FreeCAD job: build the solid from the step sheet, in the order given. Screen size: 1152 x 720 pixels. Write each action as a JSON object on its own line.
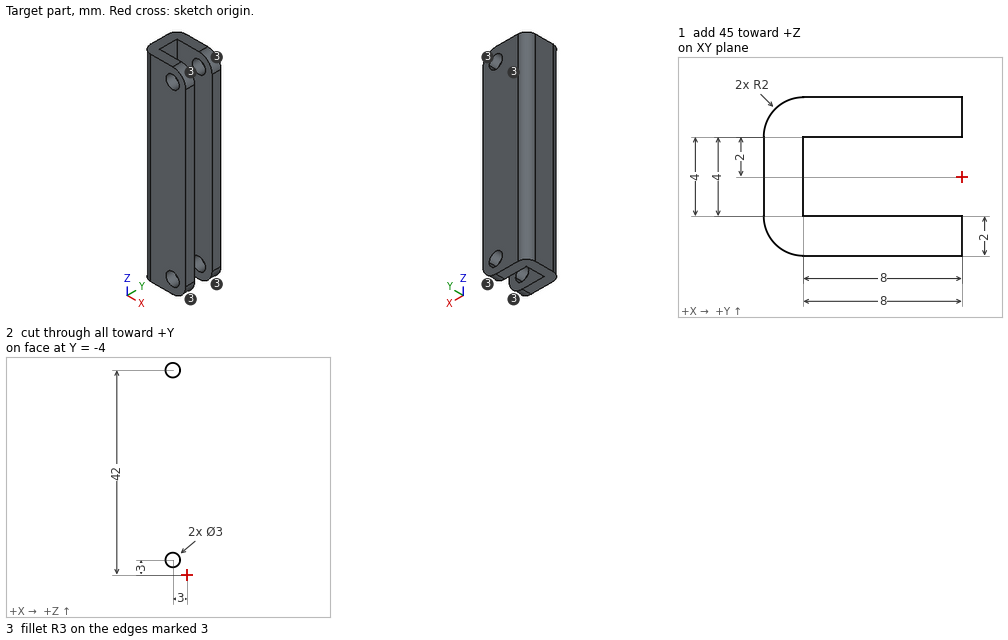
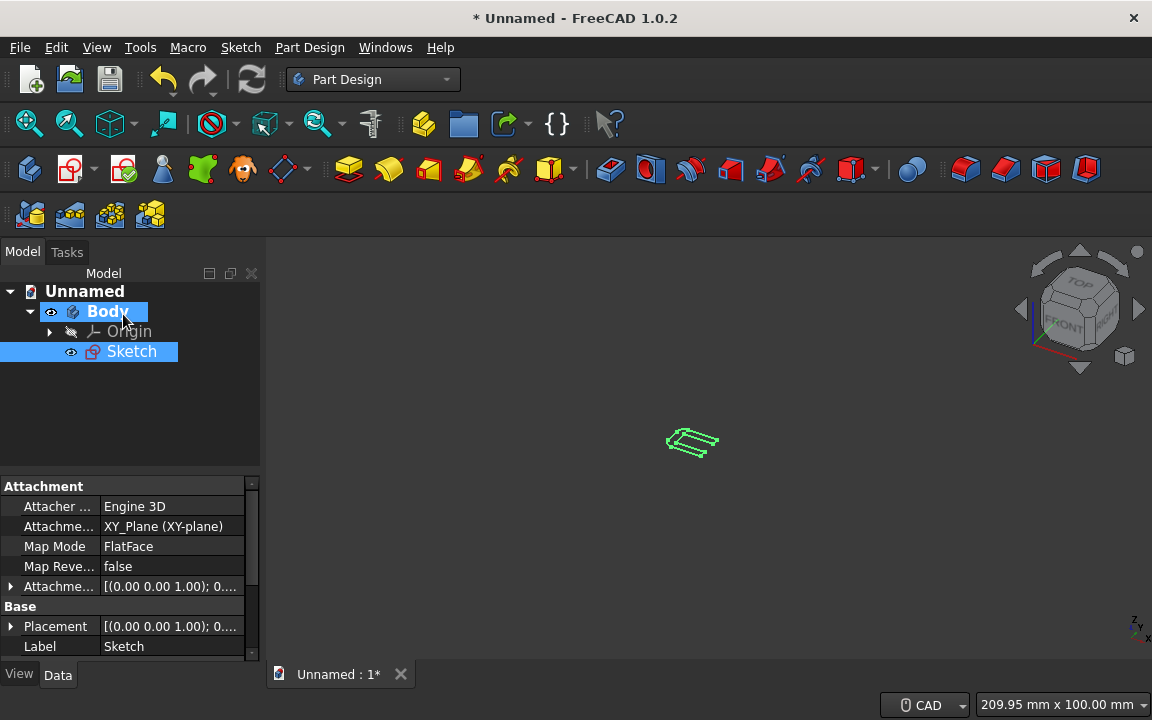
{"action": "left_click", "coordinate": [350, 170]}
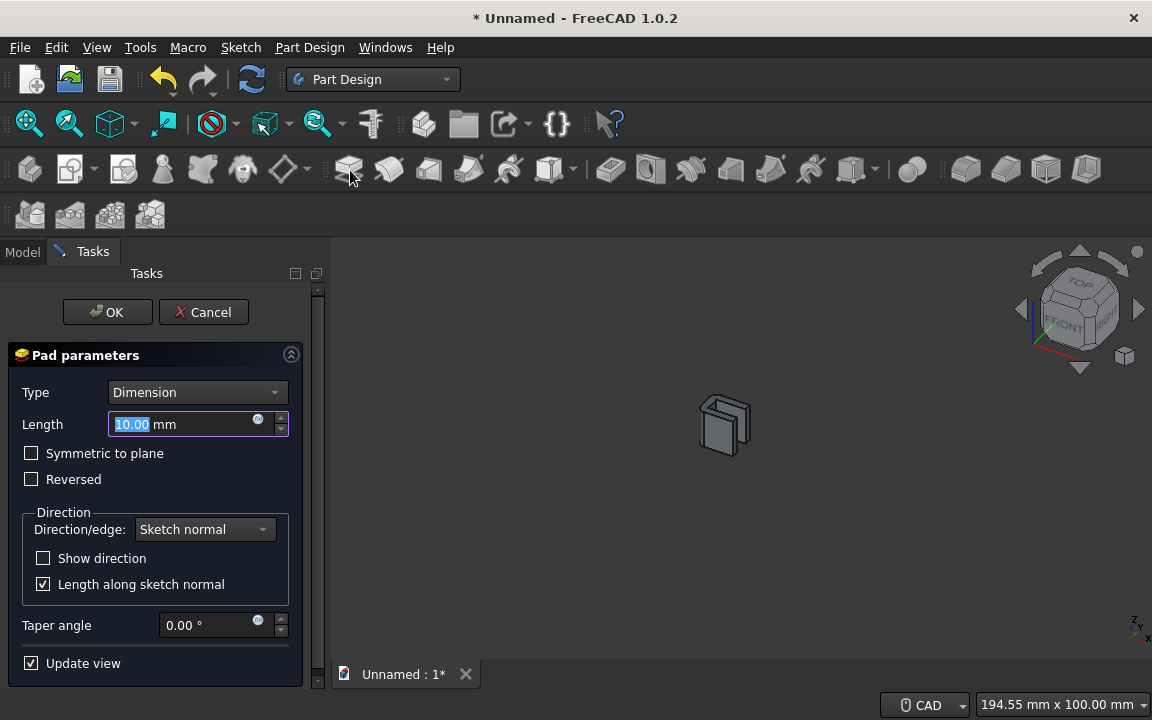
{"action": "type", "text": "45"}
{"action": "key", "text": "Tab"}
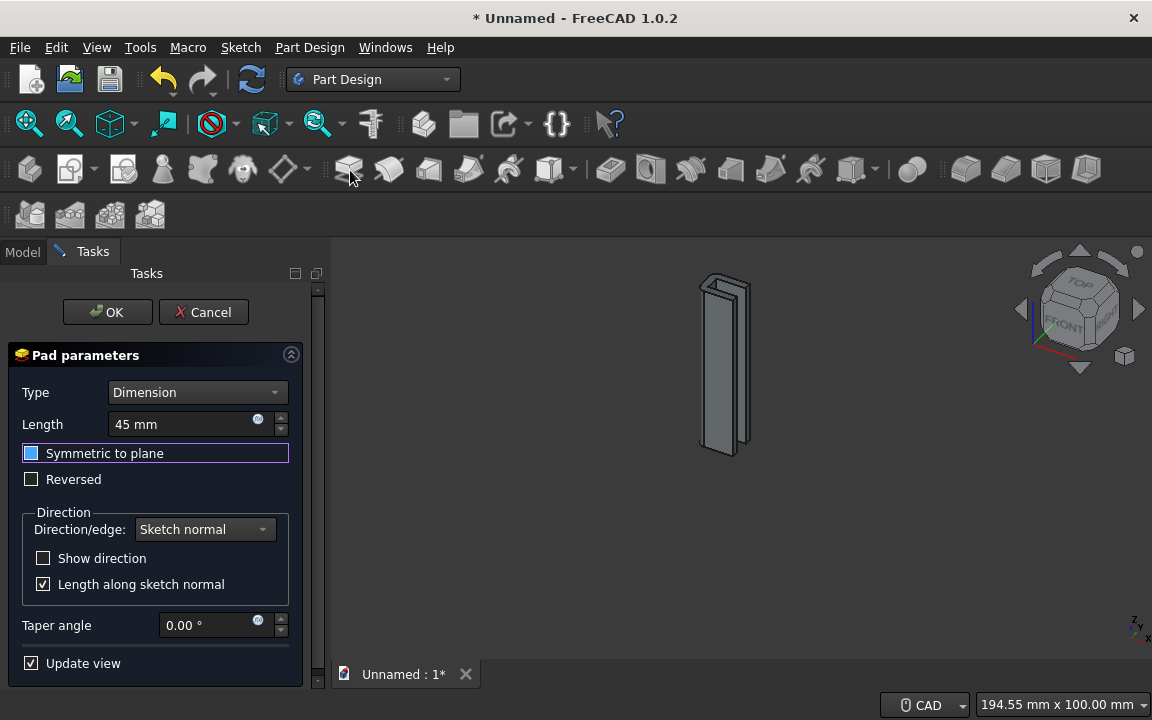
{"action": "left_click", "coordinate": [108, 312]}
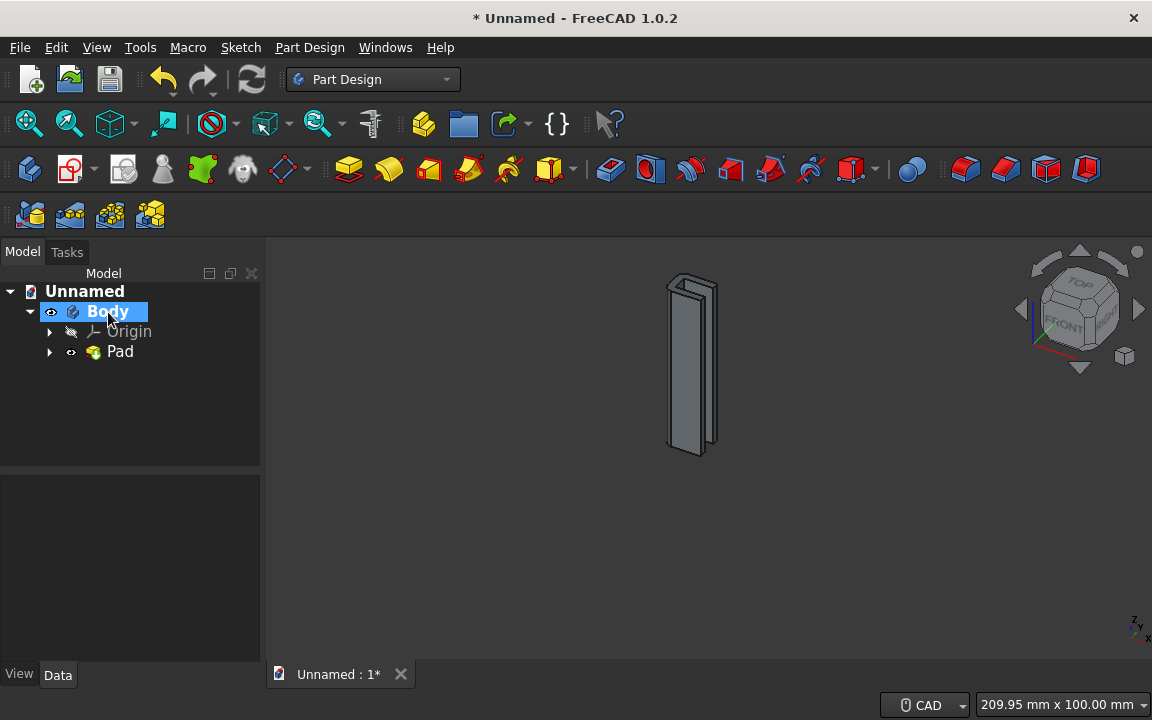
{"action": "left_click", "coordinate": [30, 124]}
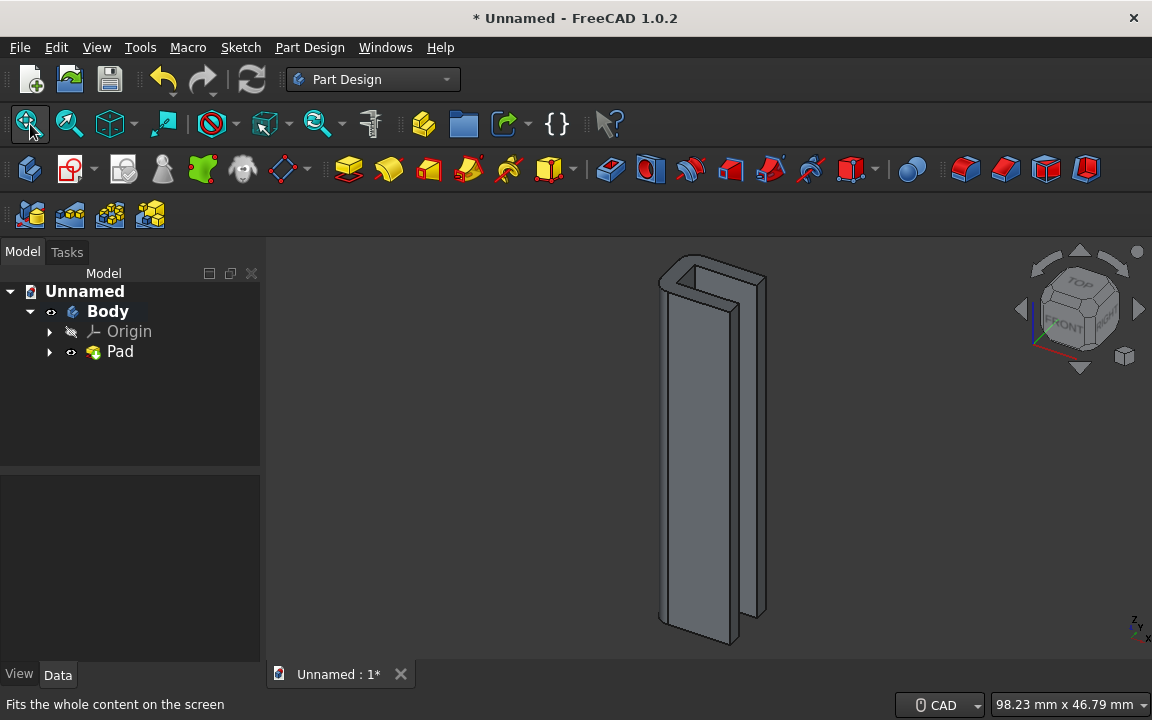
{"action": "left_click", "coordinate": [699, 373]}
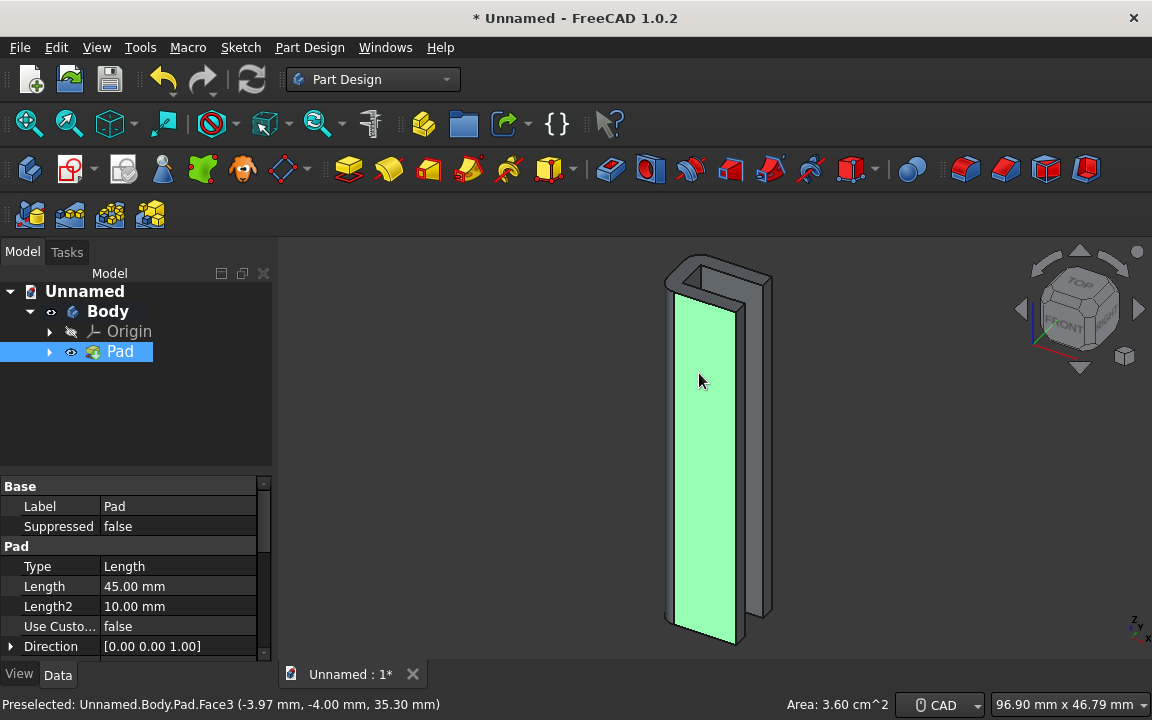
{"action": "left_click", "coordinate": [70, 170]}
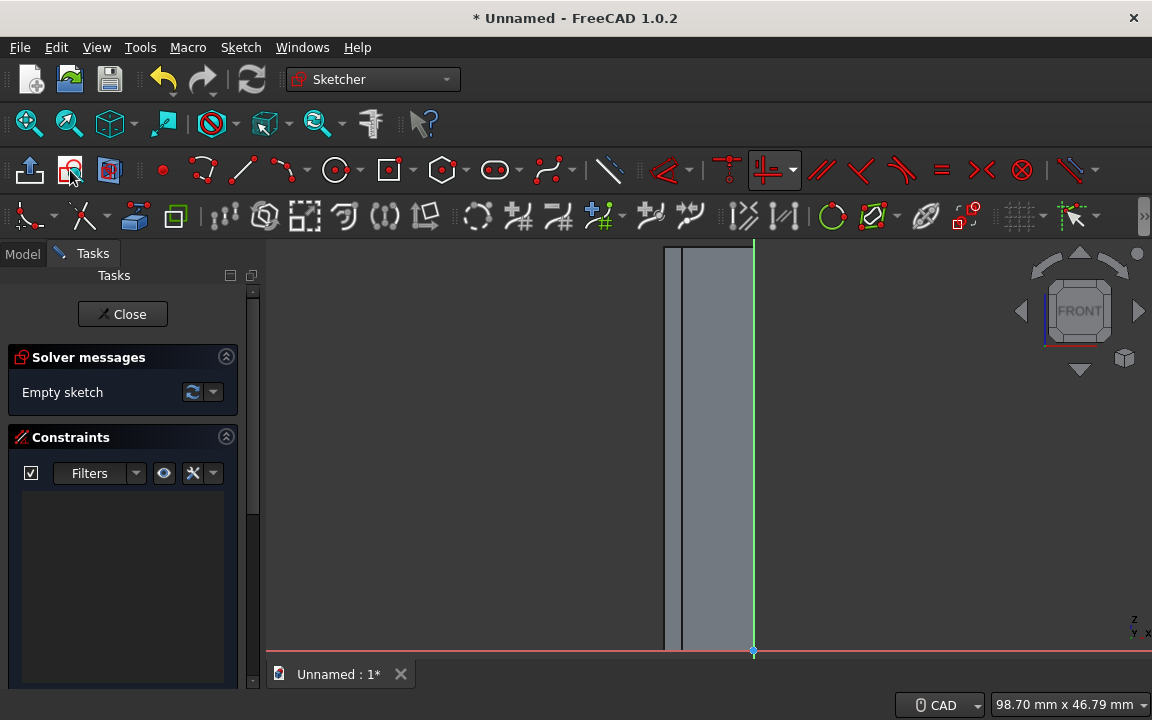
{"action": "scroll", "coordinate": [451, 435], "scroll_direction": "down", "scroll_amount": 2}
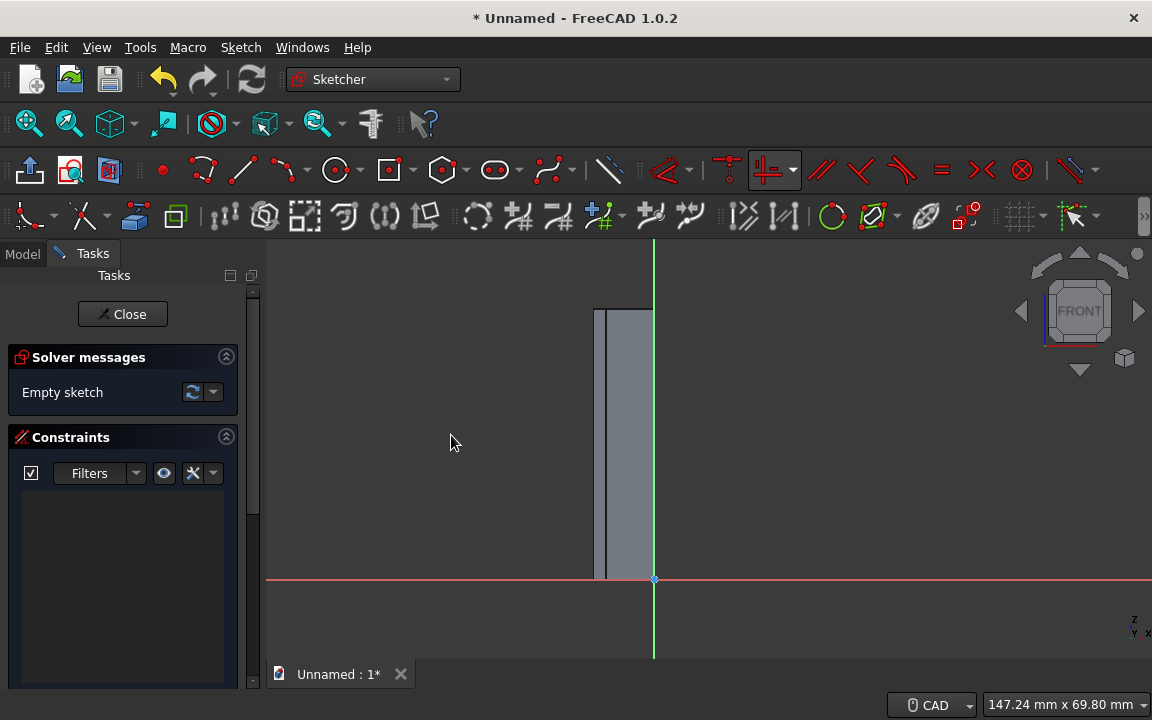
{"action": "left_click", "coordinate": [336, 170]}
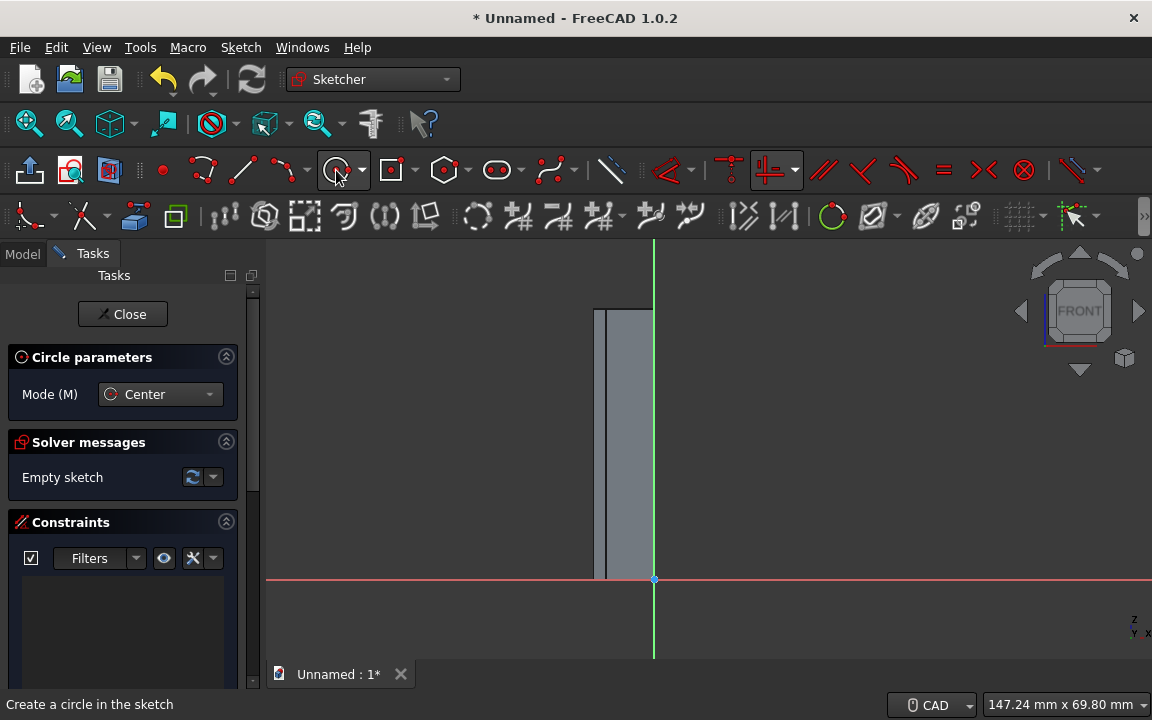
{"action": "scroll", "coordinate": [636, 562], "scroll_direction": "up", "scroll_amount": 5}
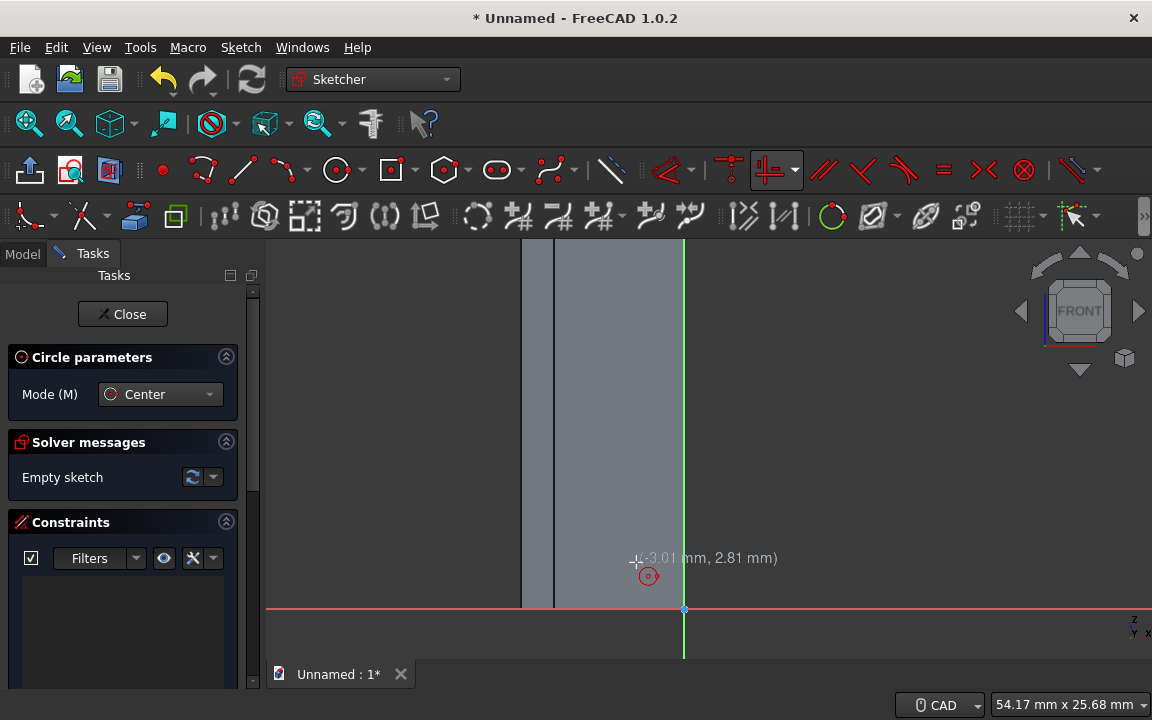
{"action": "left_click", "coordinate": [635, 560]}
{"action": "mouse_move", "coordinate": [653, 543]}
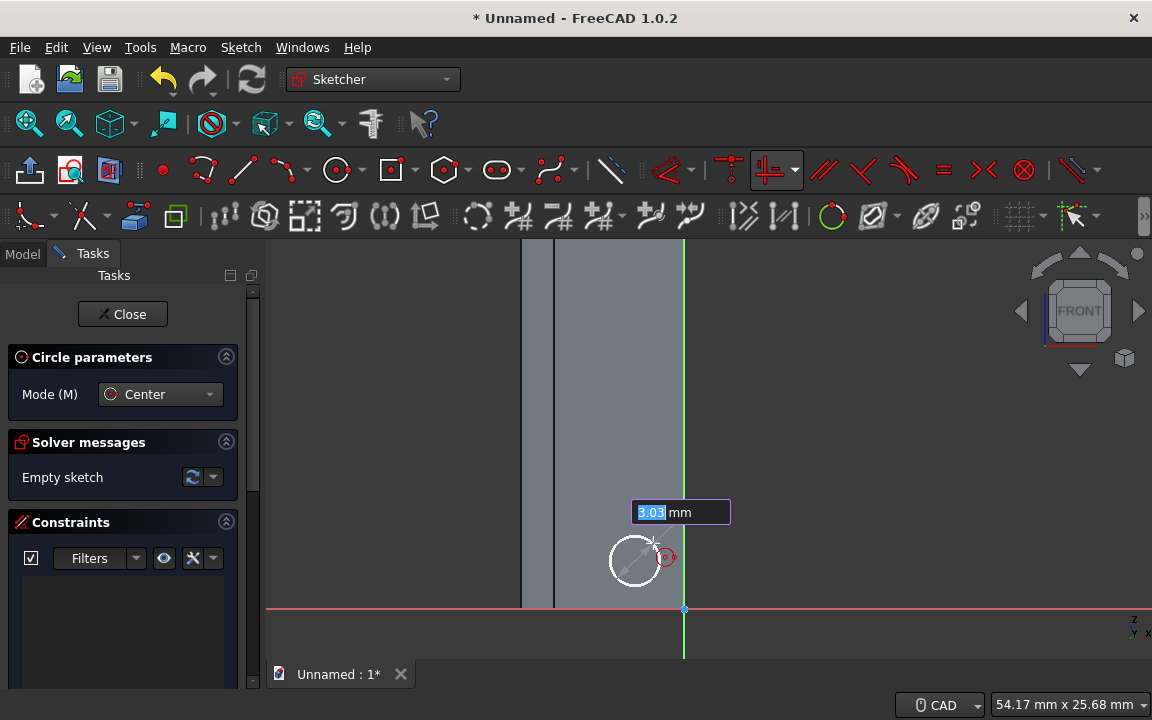
{"action": "type", "text": "3"}
{"action": "key", "text": "Return"}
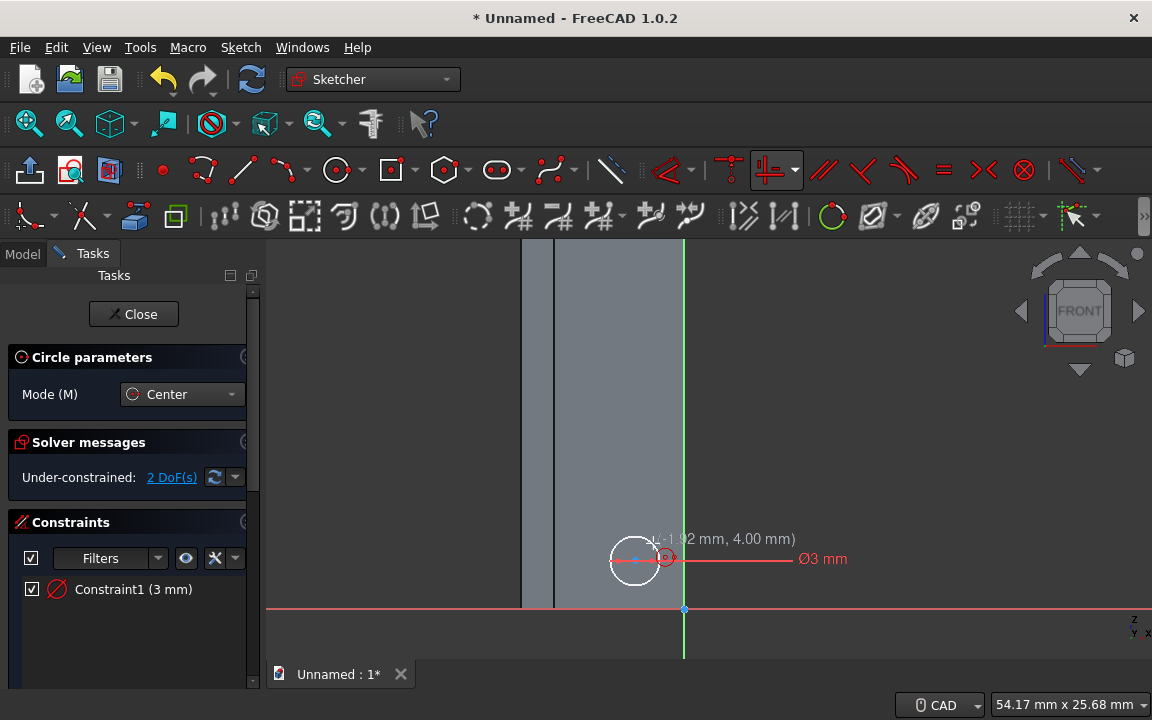
{"action": "scroll", "coordinate": [636, 563], "scroll_direction": "down", "scroll_amount": 5}